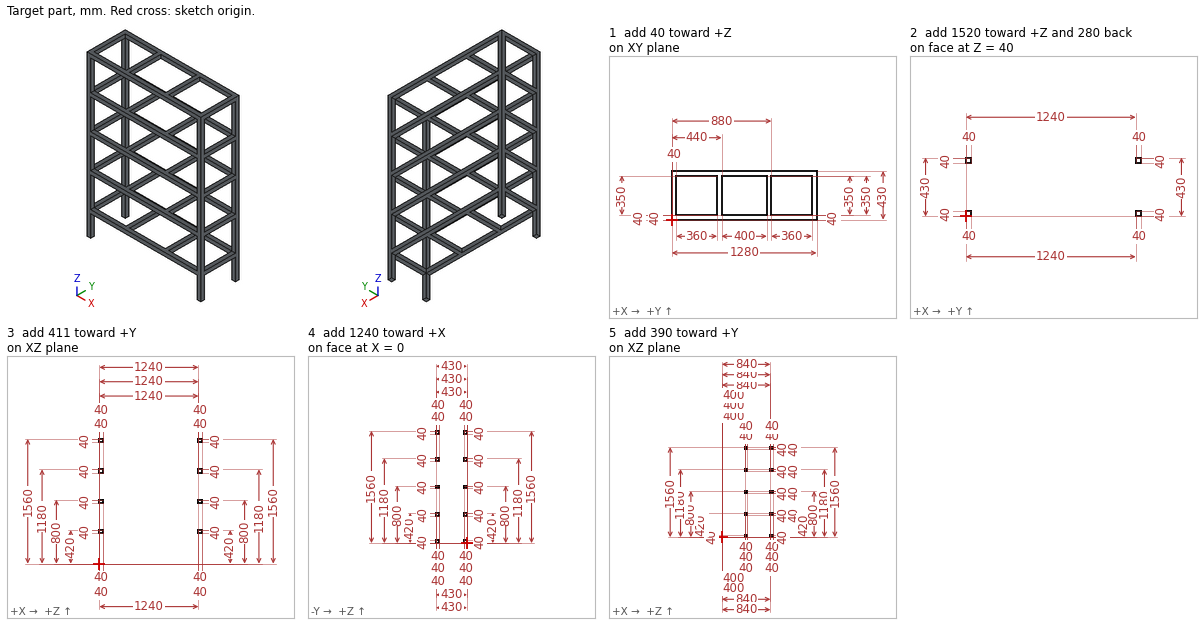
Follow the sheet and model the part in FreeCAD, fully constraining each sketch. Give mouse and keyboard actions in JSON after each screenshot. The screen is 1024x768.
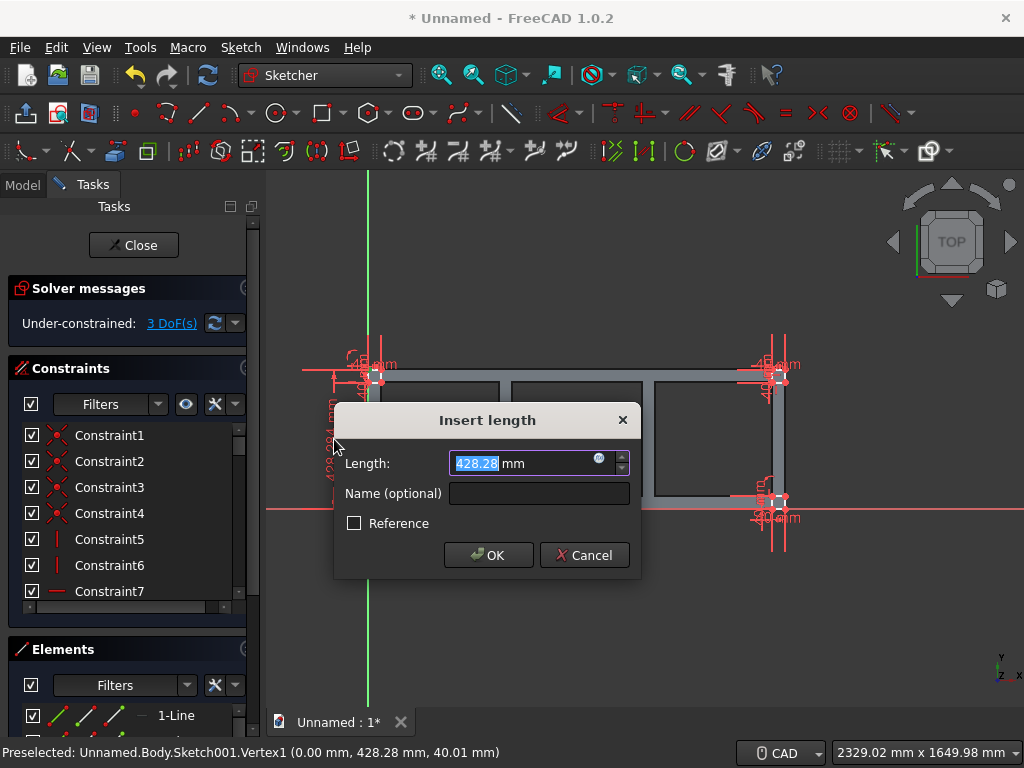
{"action": "type", "text": "430"}
{"action": "key", "text": "Return"}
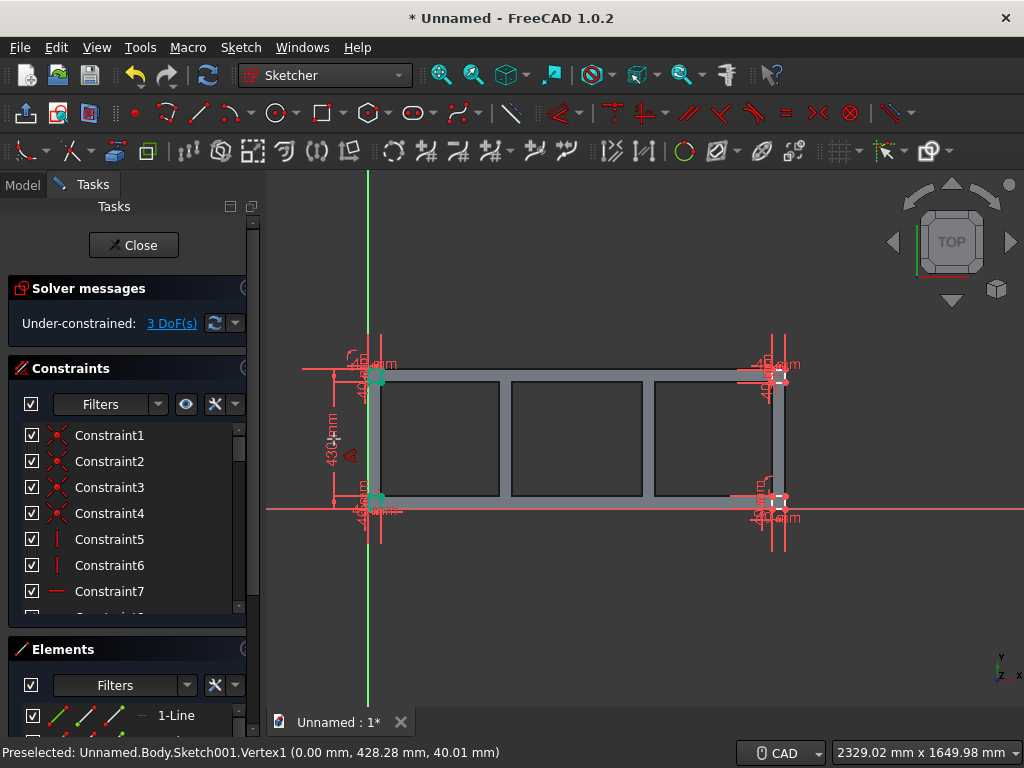
{"action": "left_click", "coordinate": [772, 370]}
{"action": "left_click", "coordinate": [334, 407]}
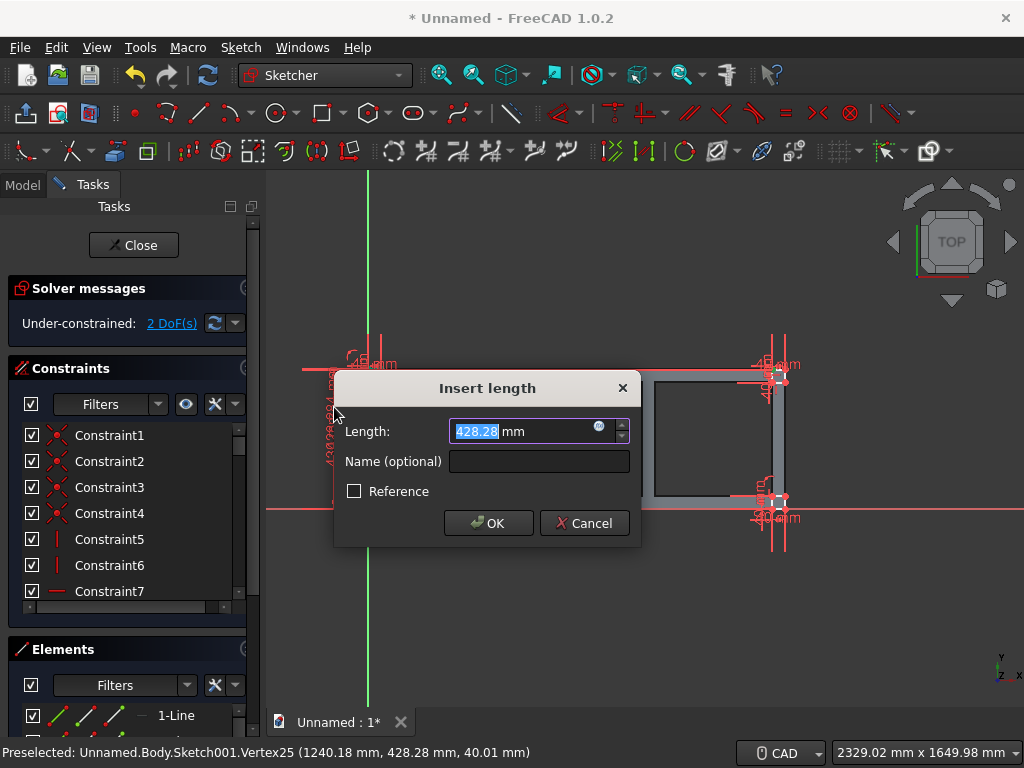
{"action": "type", "text": "430"}
{"action": "key", "text": "Return"}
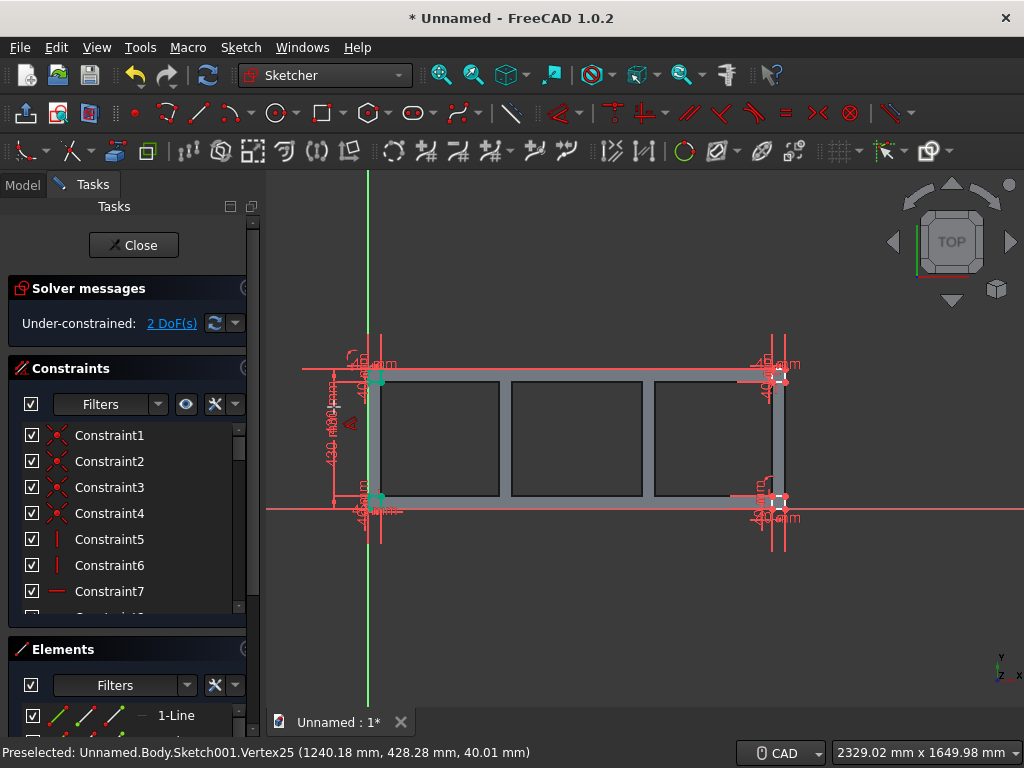
{"action": "left_click", "coordinate": [772, 496]}
{"action": "left_click", "coordinate": [570, 543]}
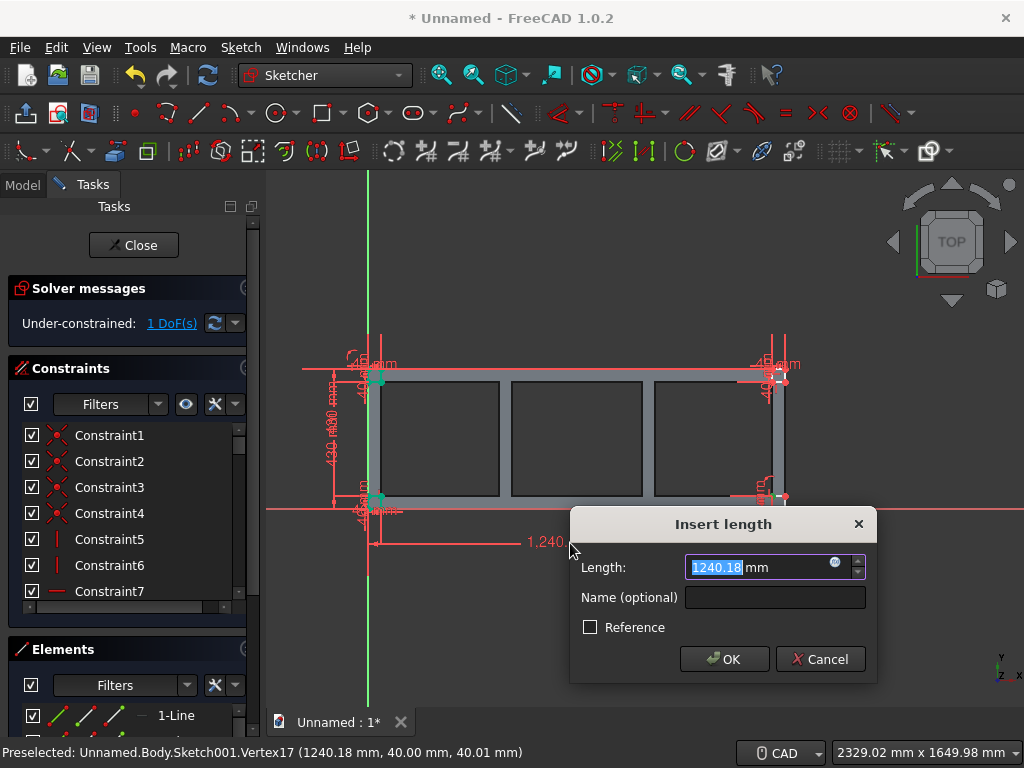
{"action": "type", "text": "1240"}
{"action": "key", "text": "Return"}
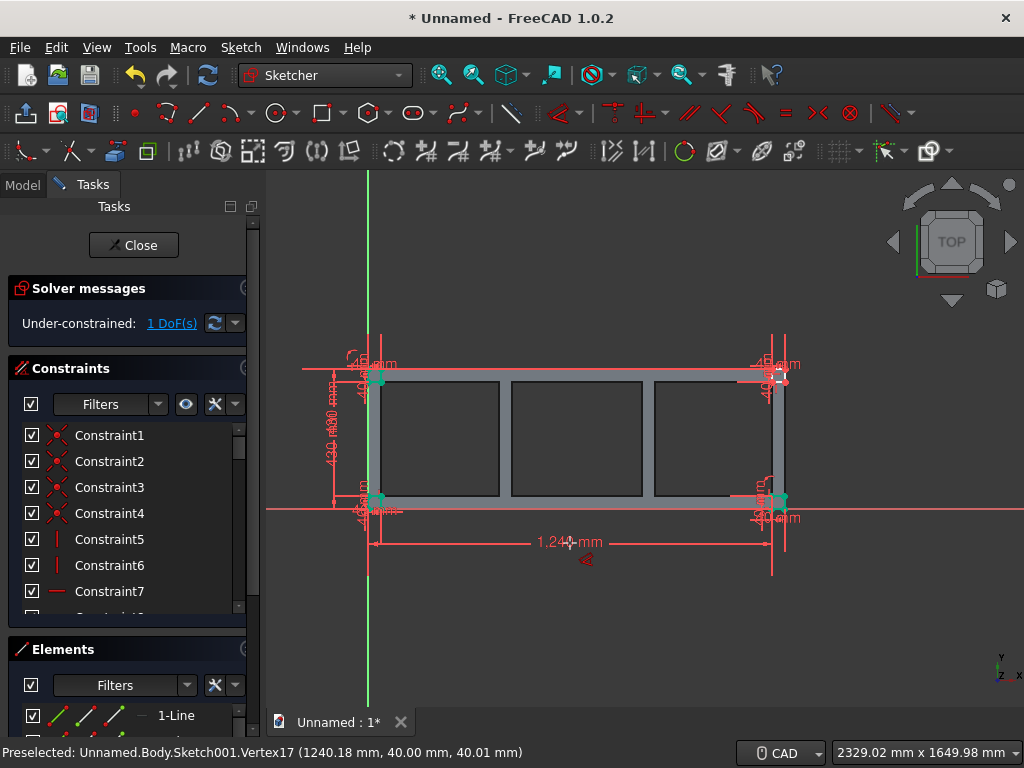
{"action": "left_click", "coordinate": [772, 369]}
{"action": "left_click", "coordinate": [477, 543]}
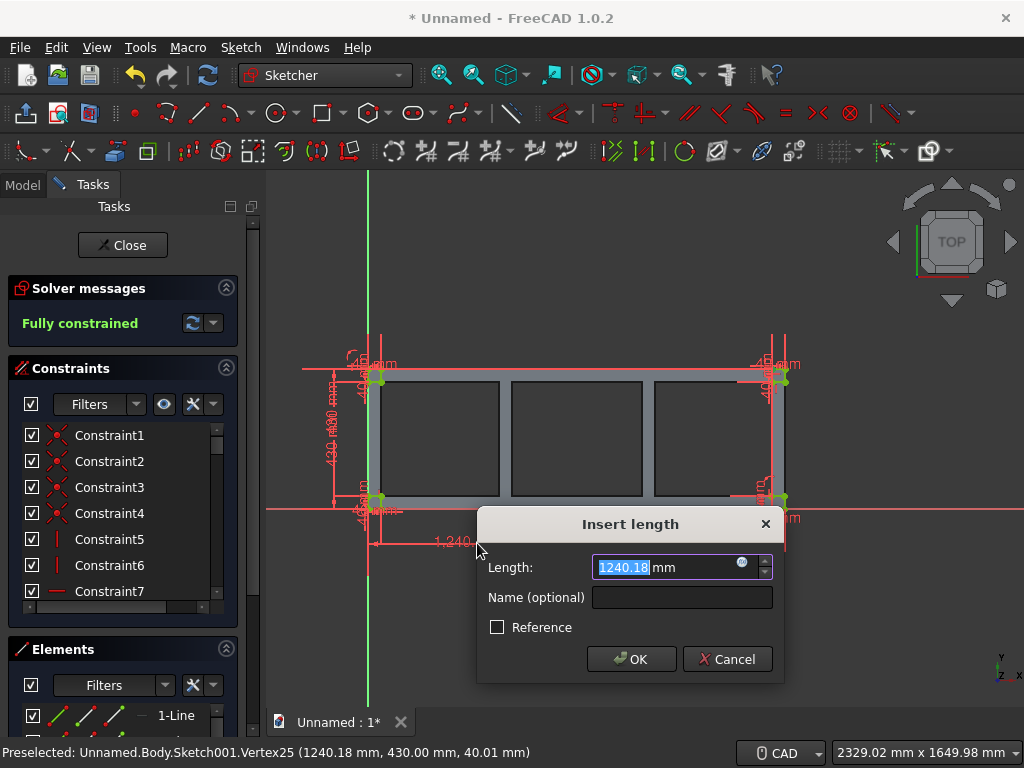
{"action": "type", "text": "1240"}
{"action": "key", "text": "Return"}
{"action": "key", "text": "Escape"}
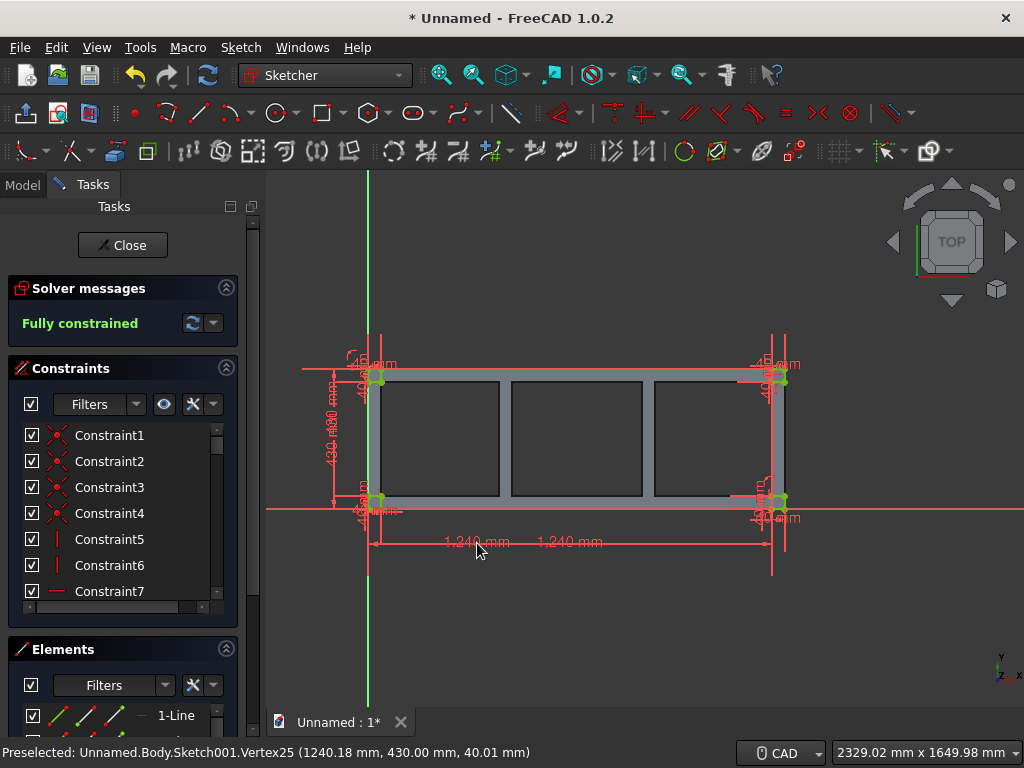
{"action": "left_click", "coordinate": [123, 245]}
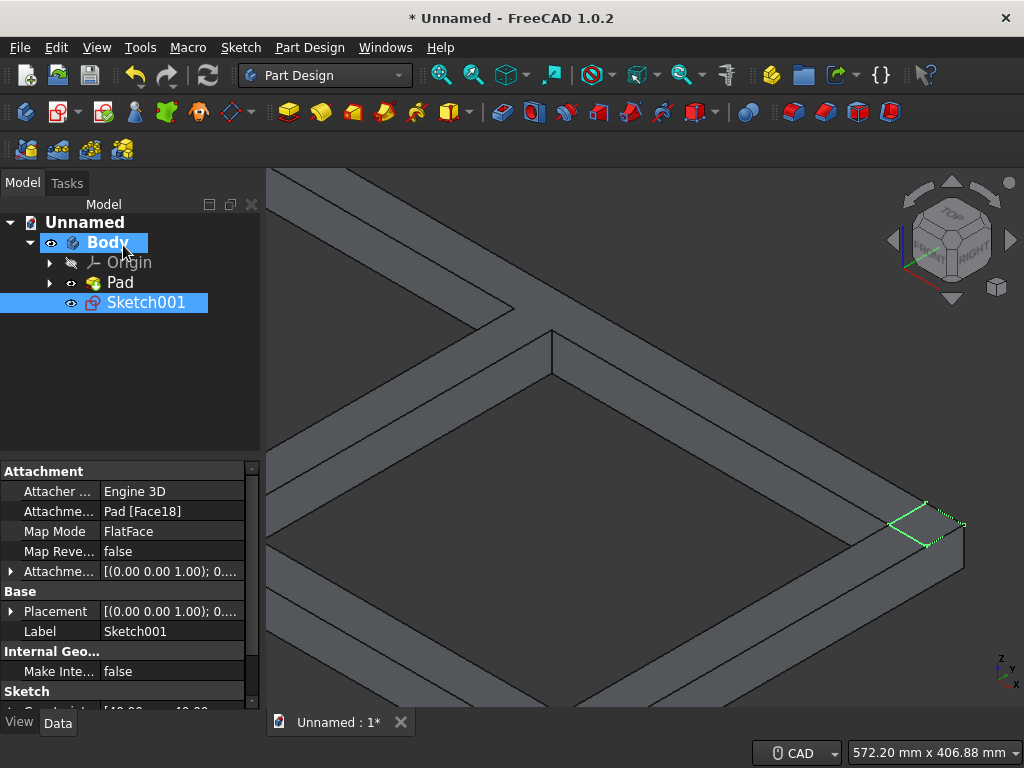
{"action": "left_click", "coordinate": [290, 112]}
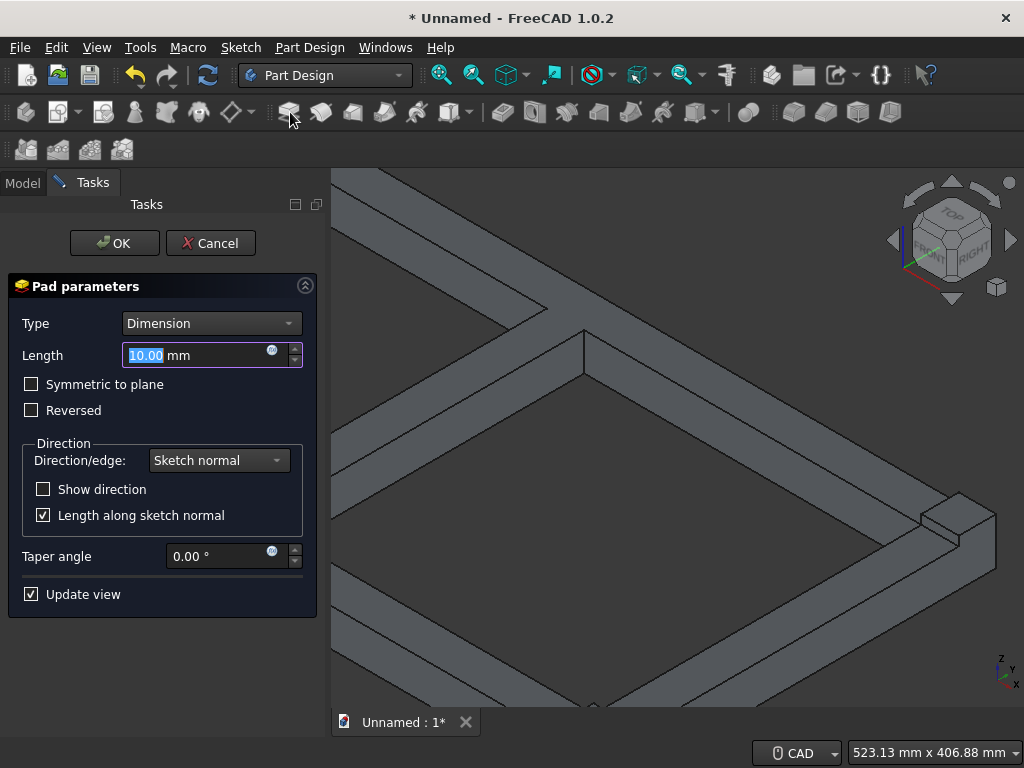
{"action": "left_click", "coordinate": [212, 324]}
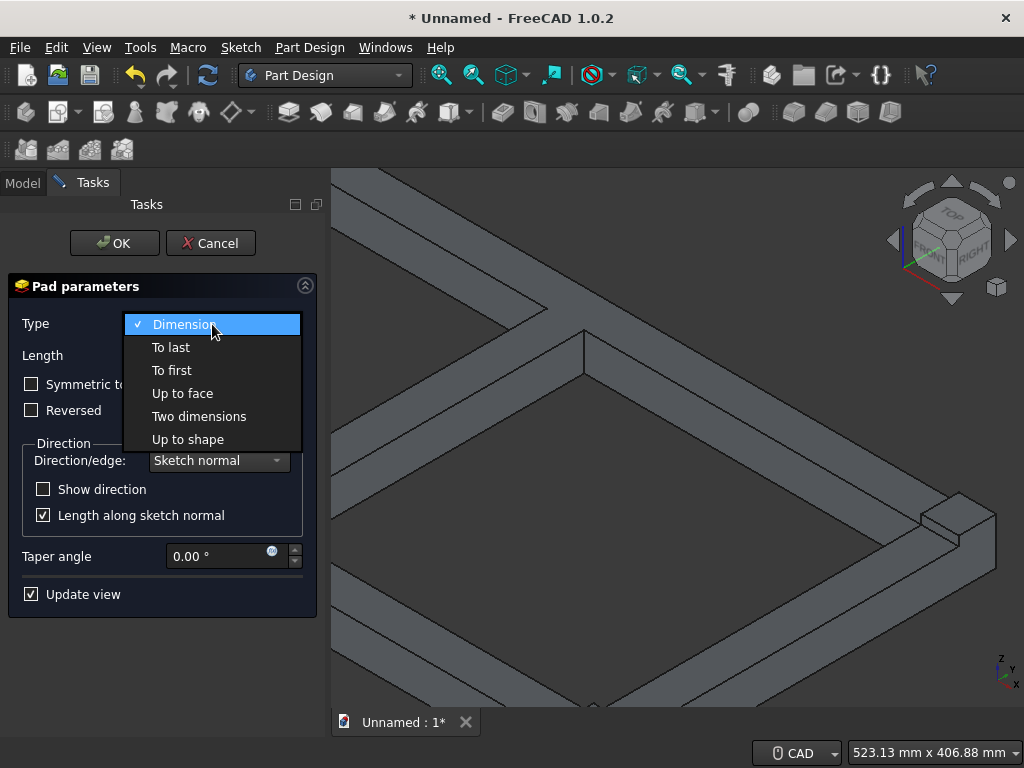
{"action": "left_click", "coordinate": [212, 416]}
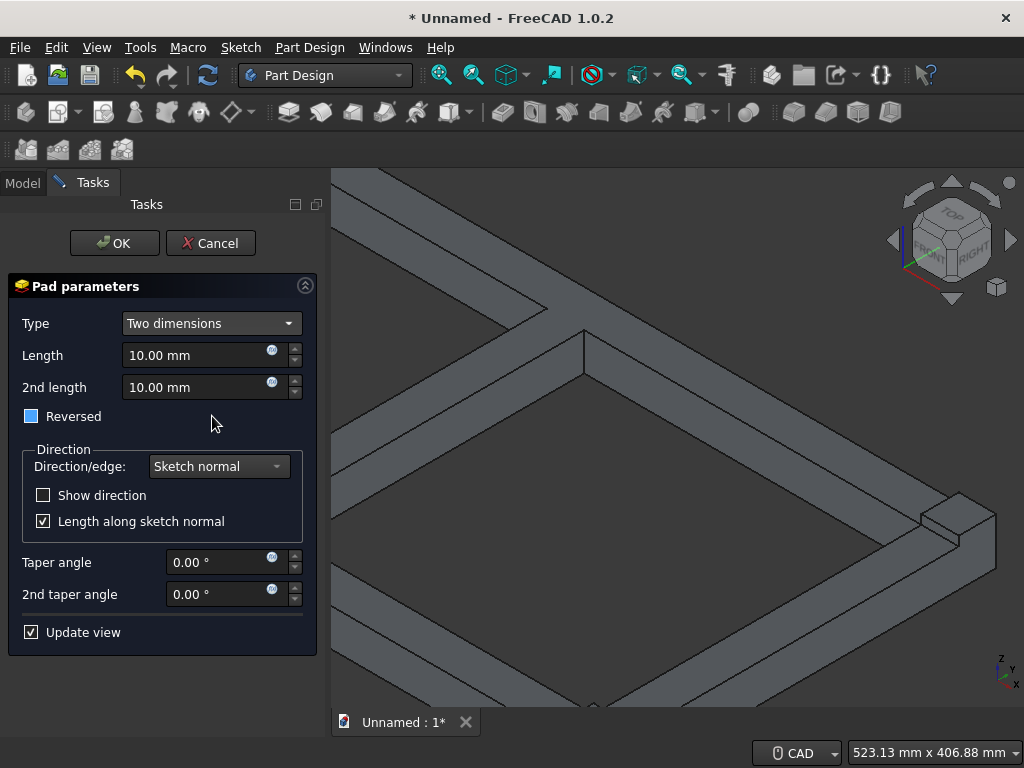
{"action": "triple_click", "coordinate": [204, 355]}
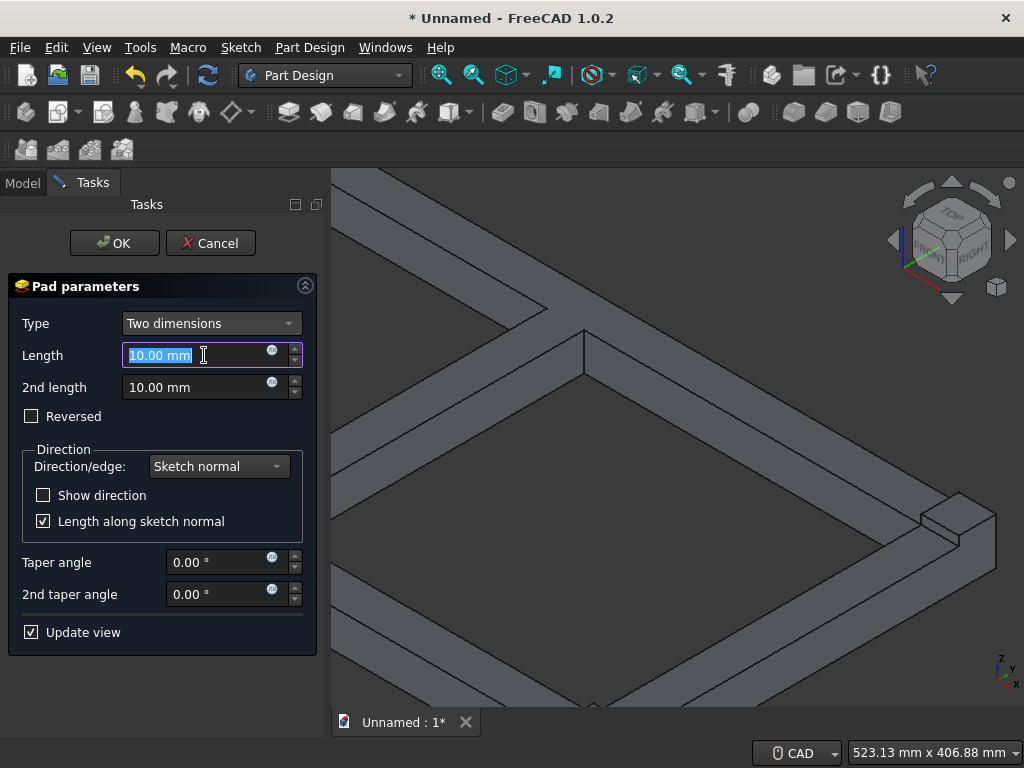
{"action": "type", "text": "1520"}
{"action": "key", "text": "Tab"}